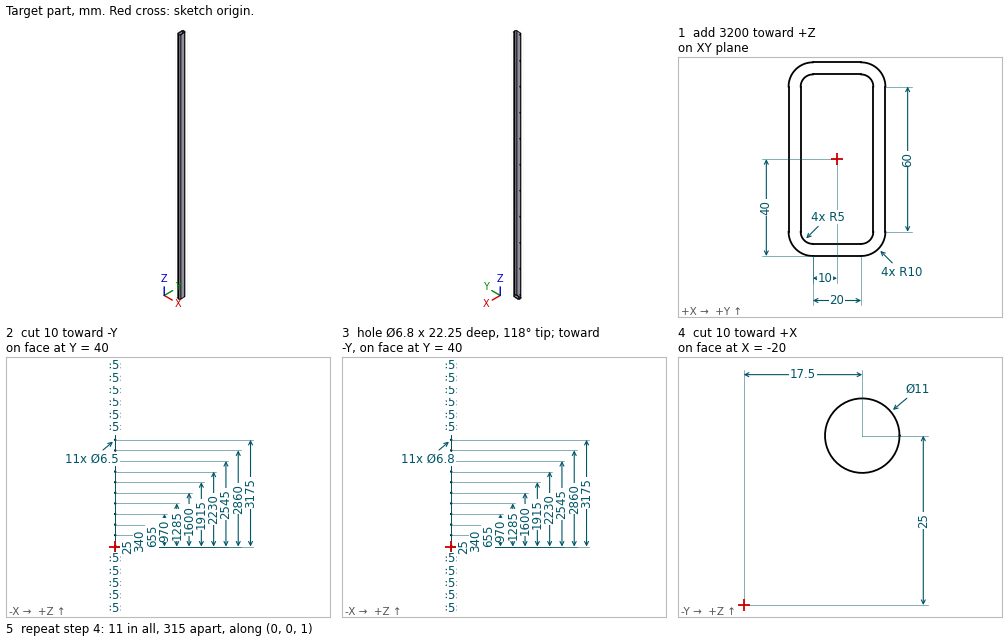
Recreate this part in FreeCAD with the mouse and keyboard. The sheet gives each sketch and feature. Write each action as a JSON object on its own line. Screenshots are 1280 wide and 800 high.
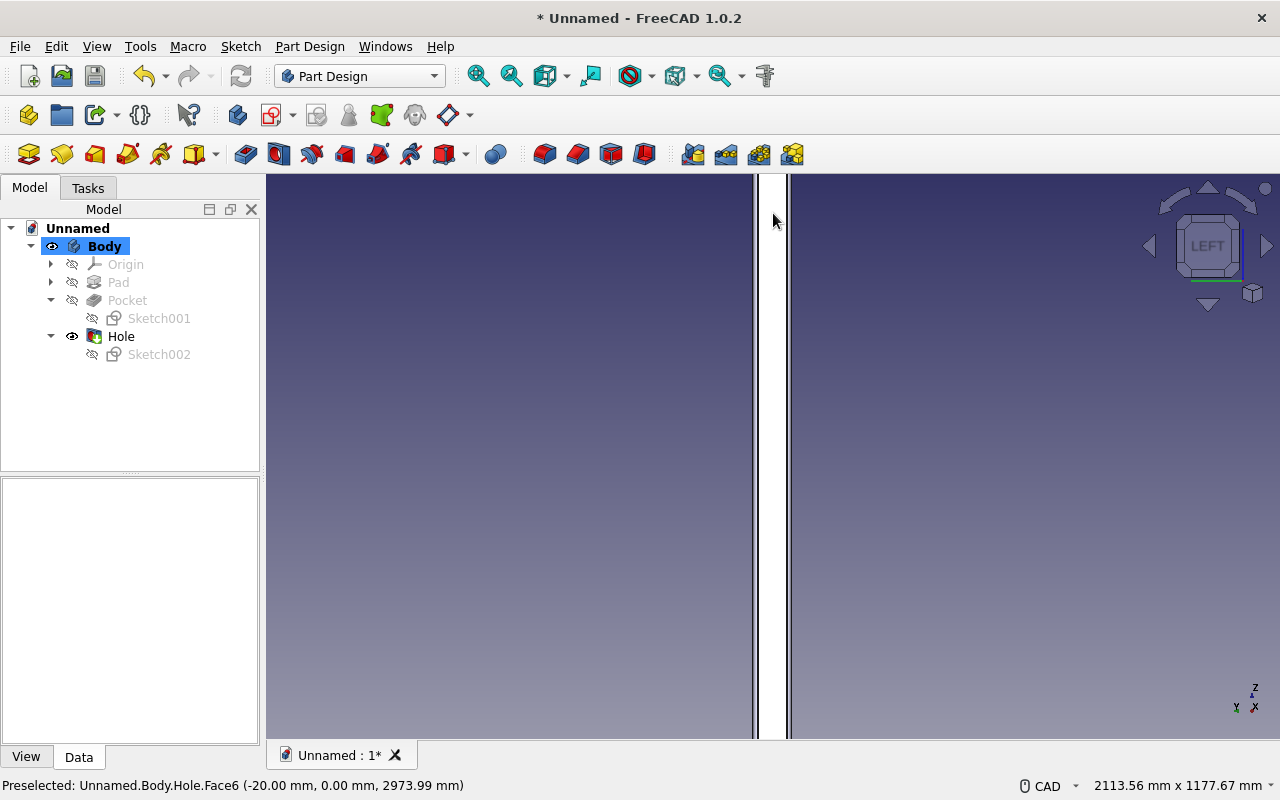
{"action": "left_click", "coordinate": [772, 216]}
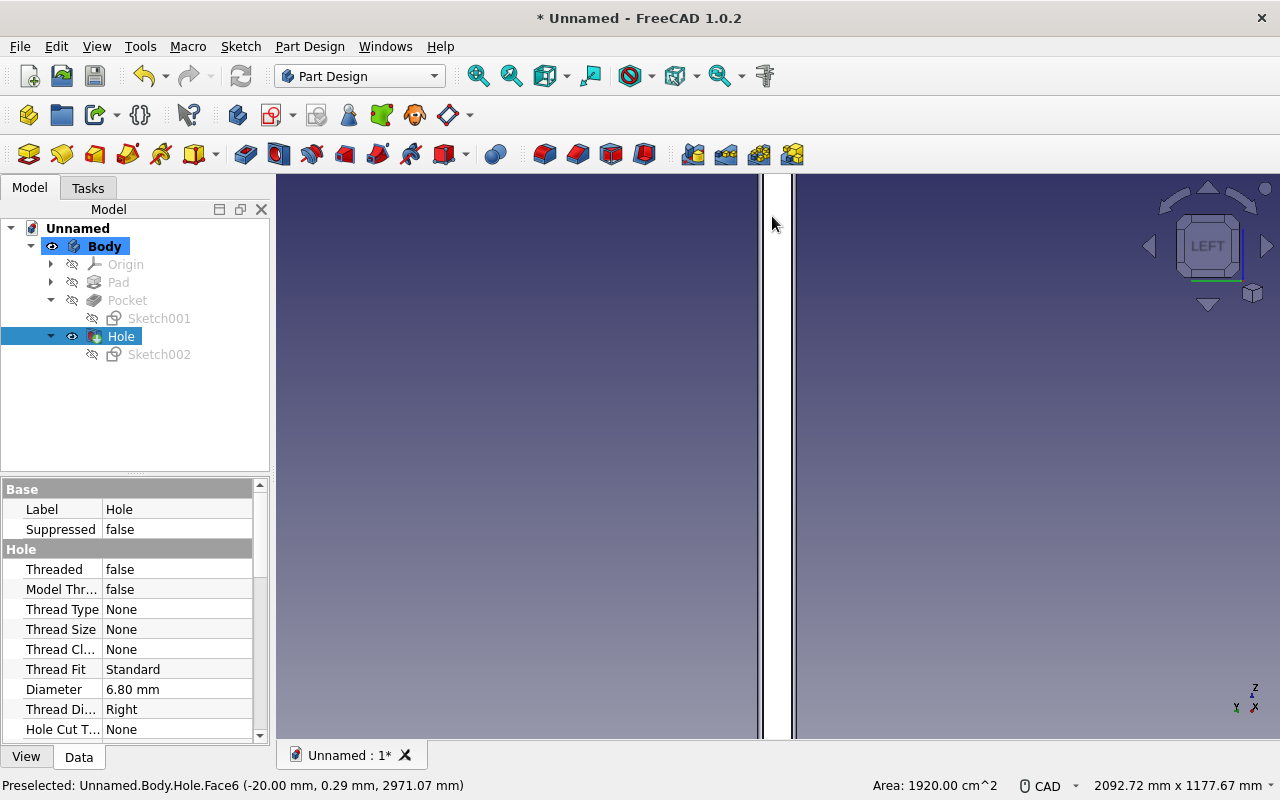
{"action": "left_click", "coordinate": [270, 116]}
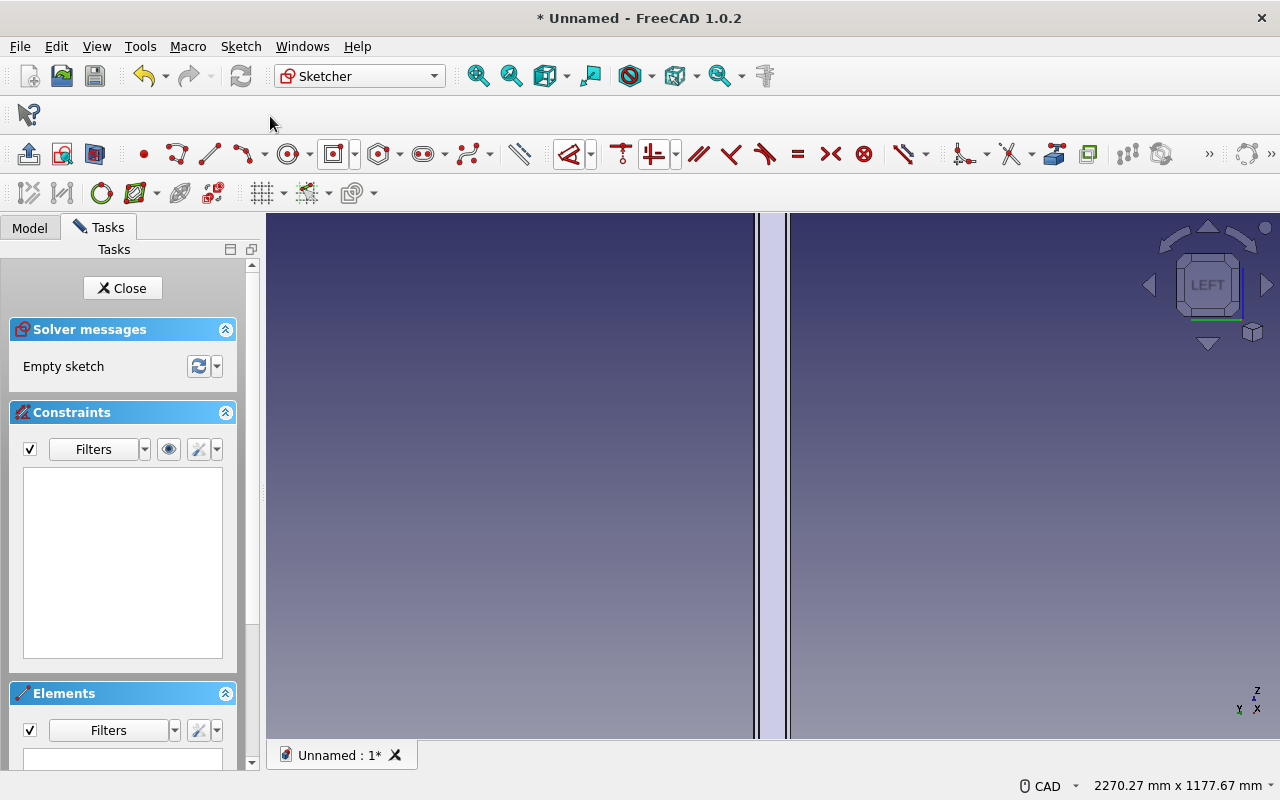
{"action": "scroll", "coordinate": [704, 476], "scroll_direction": "down", "scroll_amount": 5}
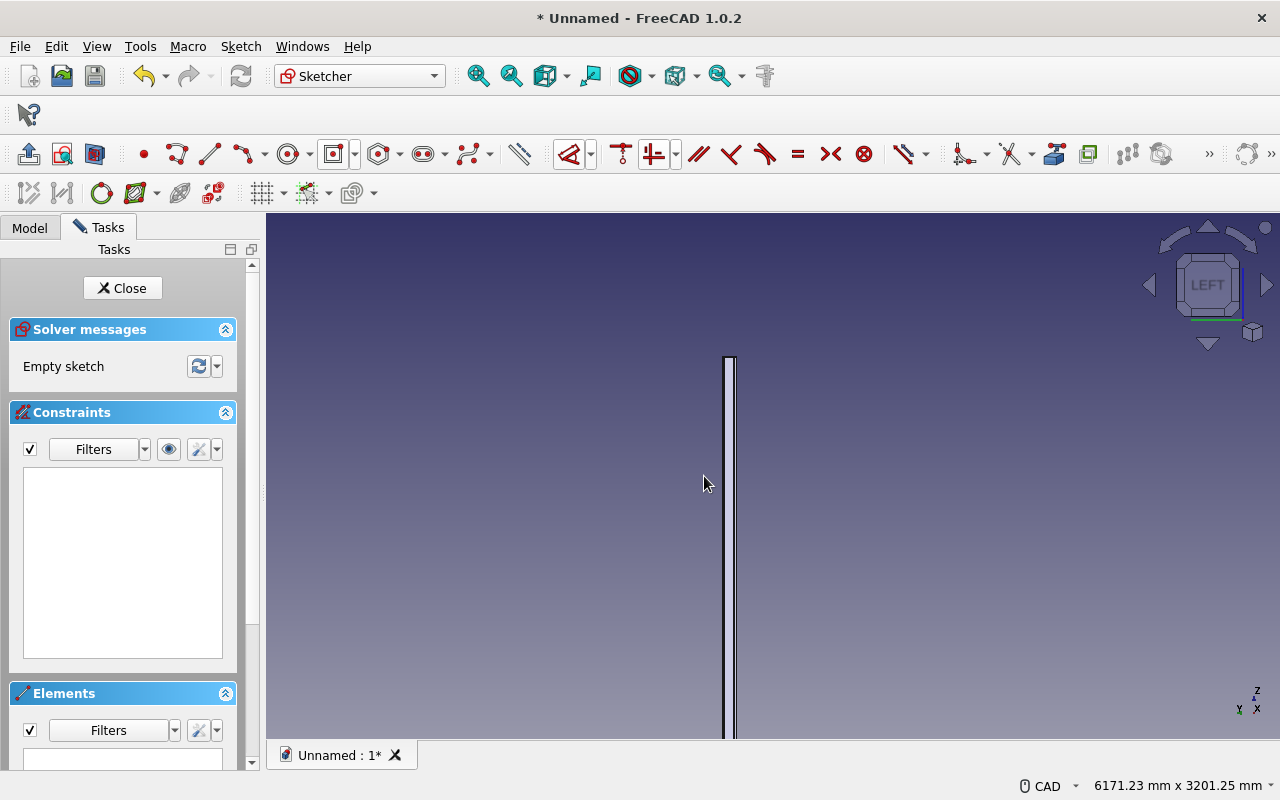
{"action": "scroll", "coordinate": [704, 476], "scroll_direction": "down", "scroll_amount": 5}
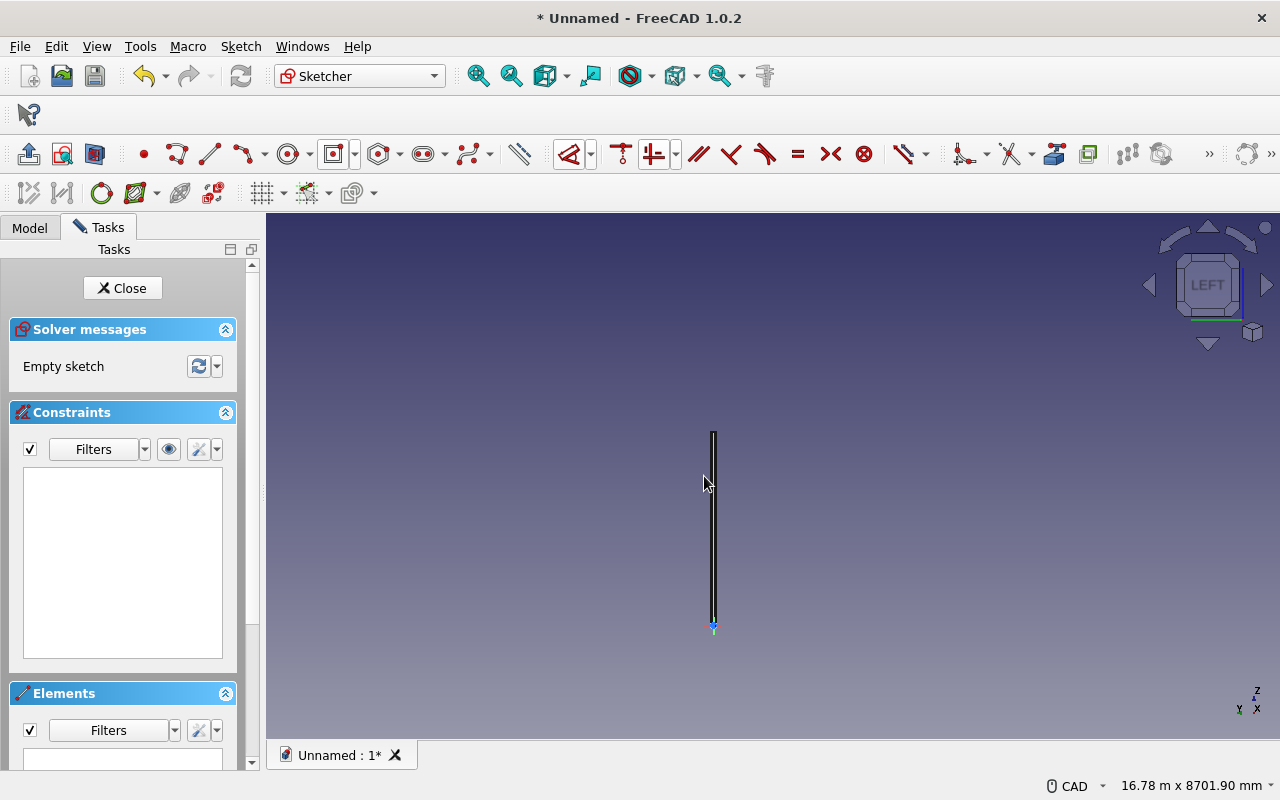
{"action": "scroll", "coordinate": [715, 632], "scroll_direction": "up", "scroll_amount": 15}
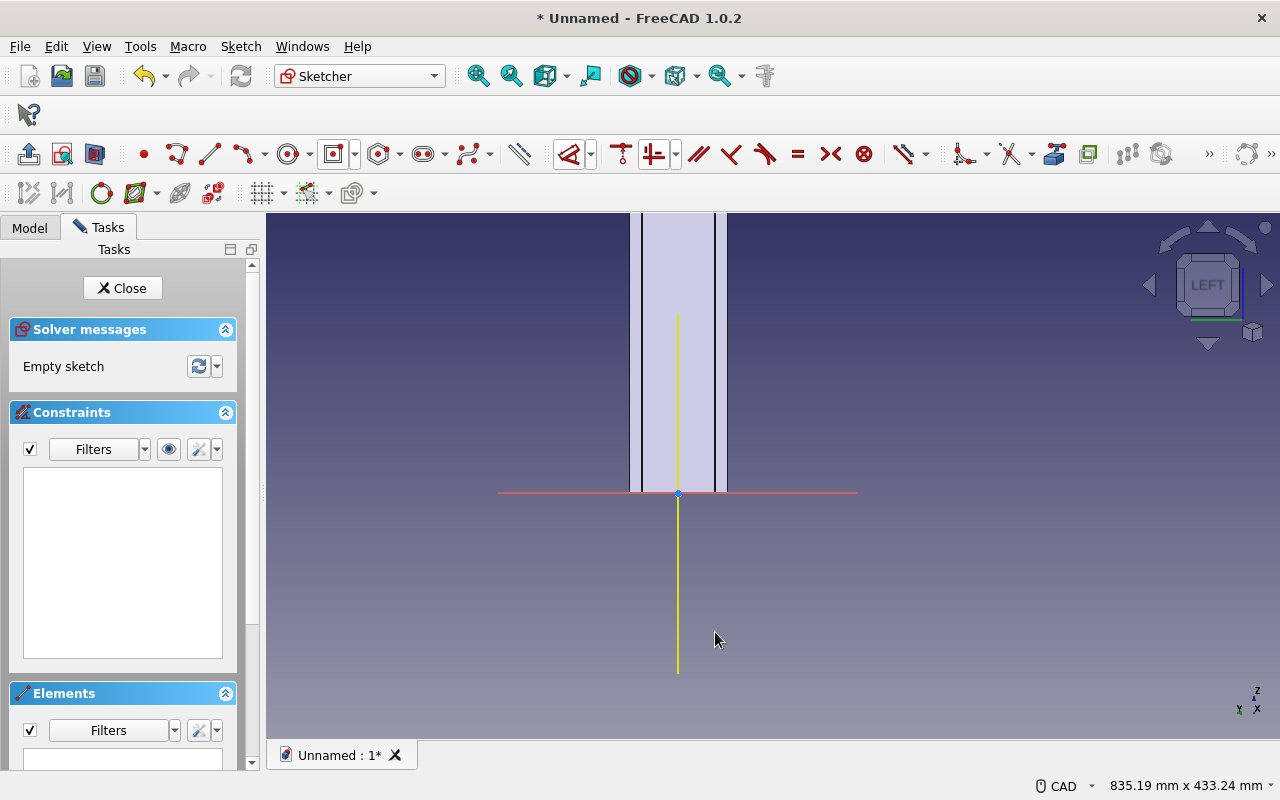
{"action": "scroll", "coordinate": [699, 462], "scroll_direction": "up", "scroll_amount": 15}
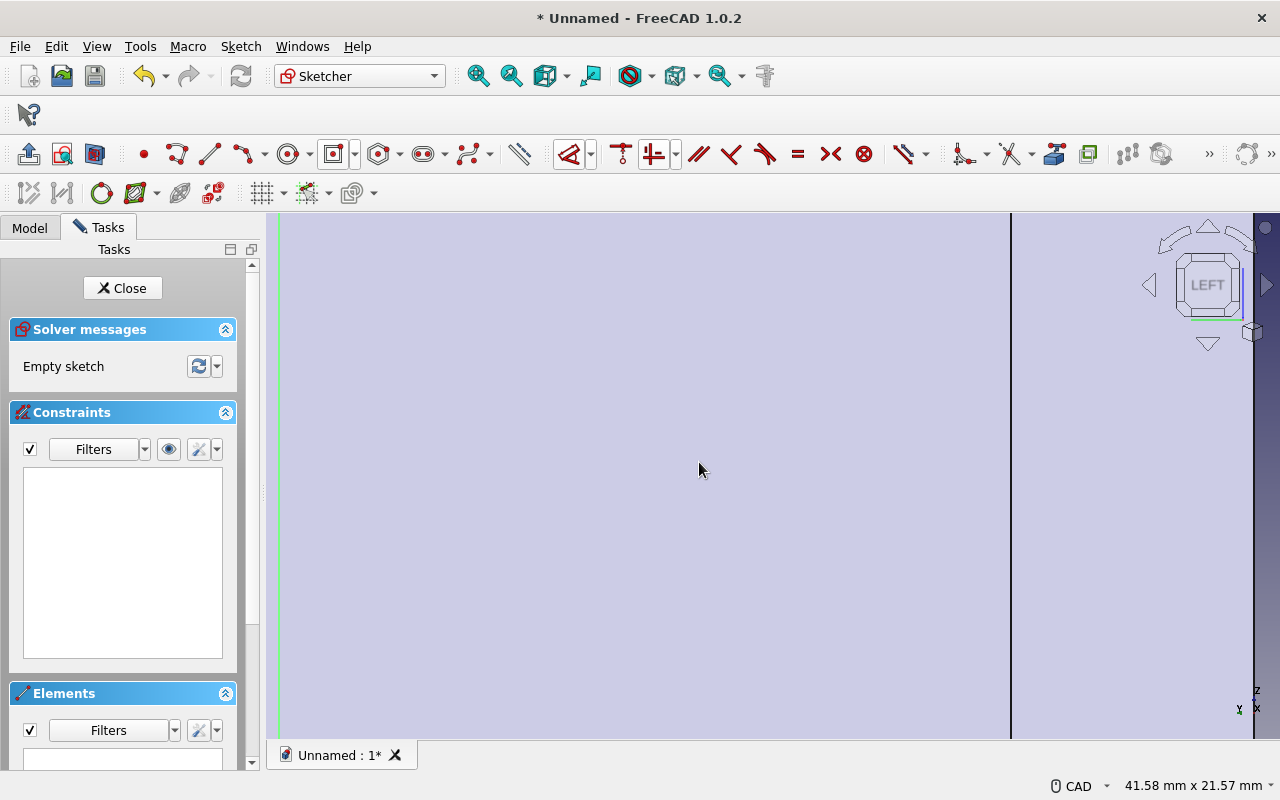
{"action": "left_click", "coordinate": [288, 154]}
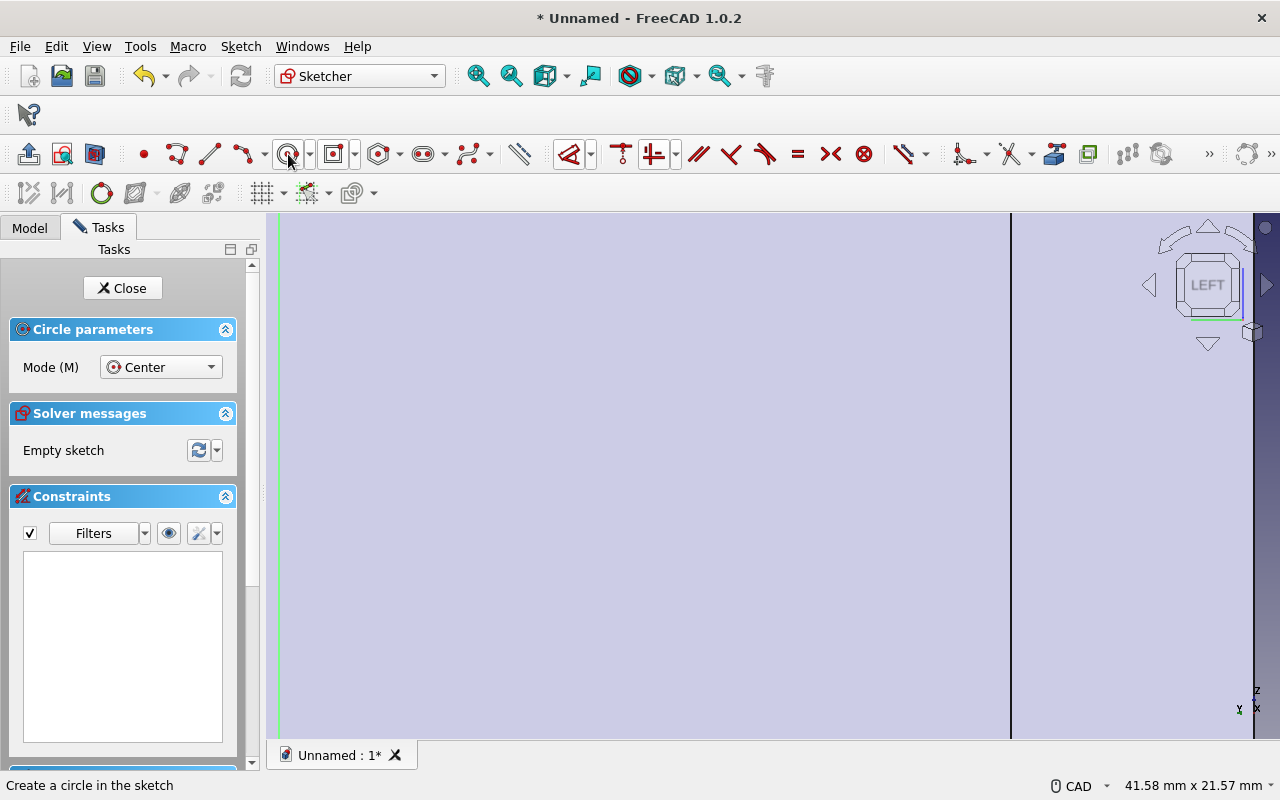
{"action": "left_click", "coordinate": [706, 470]}
{"action": "left_click", "coordinate": [801, 375]}
{"action": "key", "text": "Escape"}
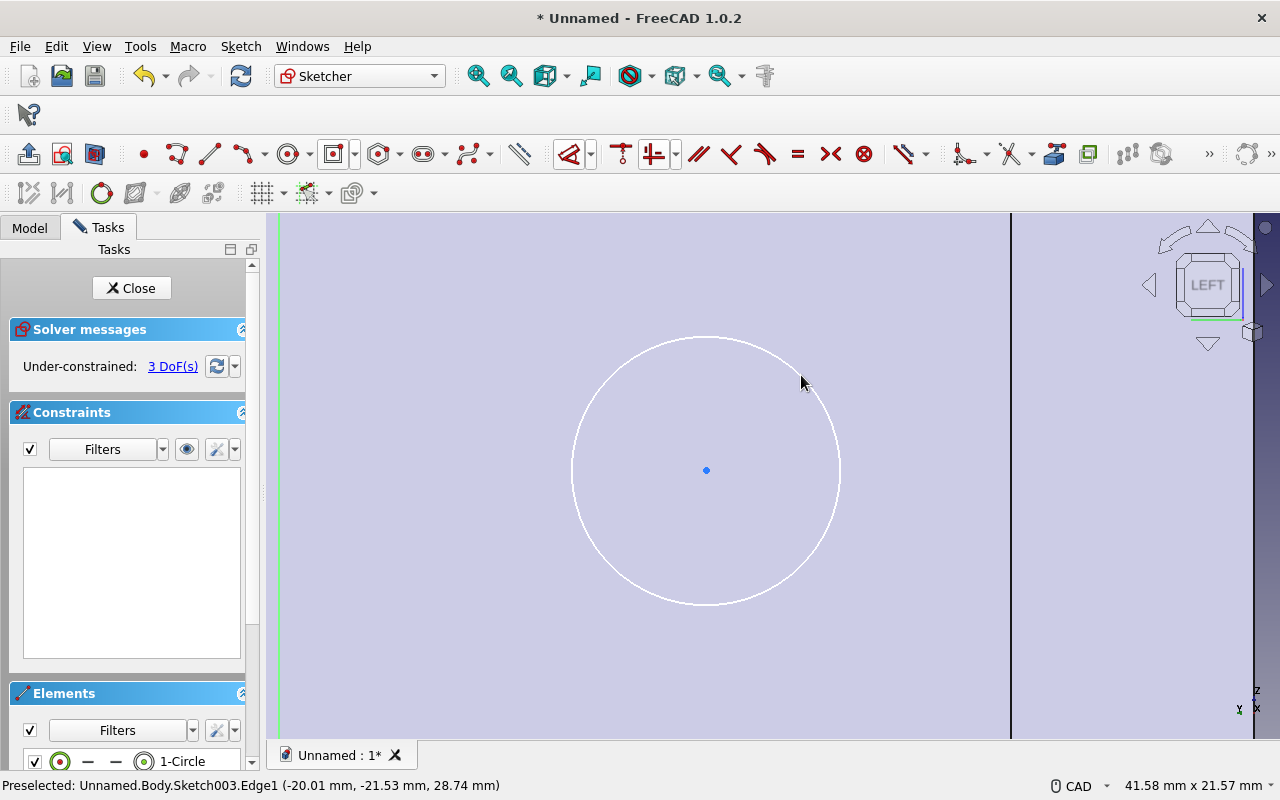
{"action": "left_click", "coordinate": [801, 376]}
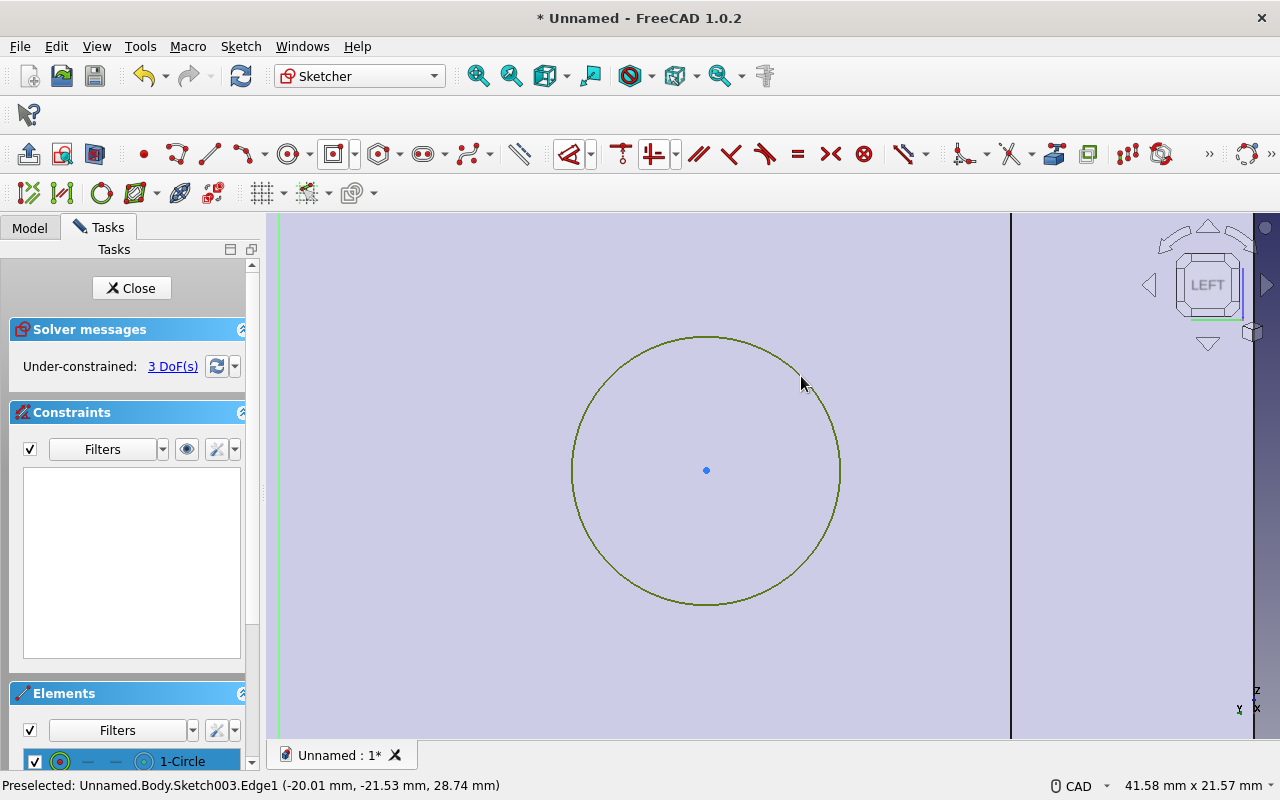
{"action": "left_click", "coordinate": [590, 154]}